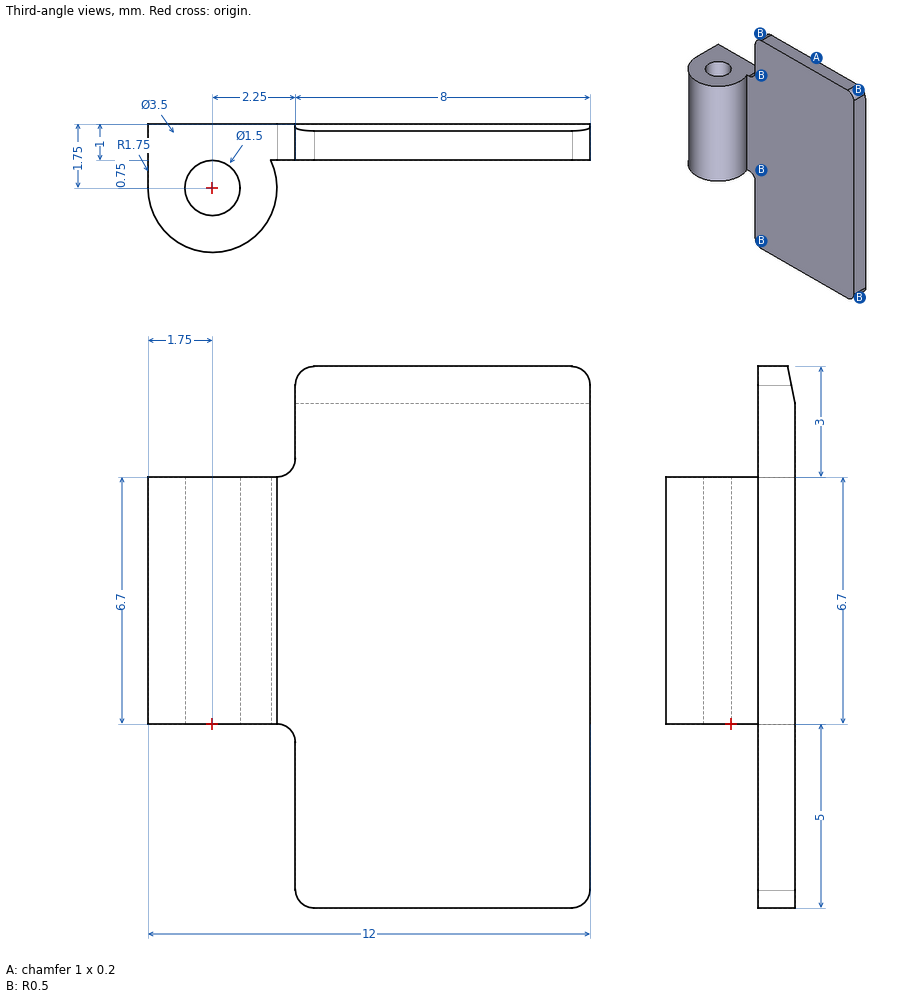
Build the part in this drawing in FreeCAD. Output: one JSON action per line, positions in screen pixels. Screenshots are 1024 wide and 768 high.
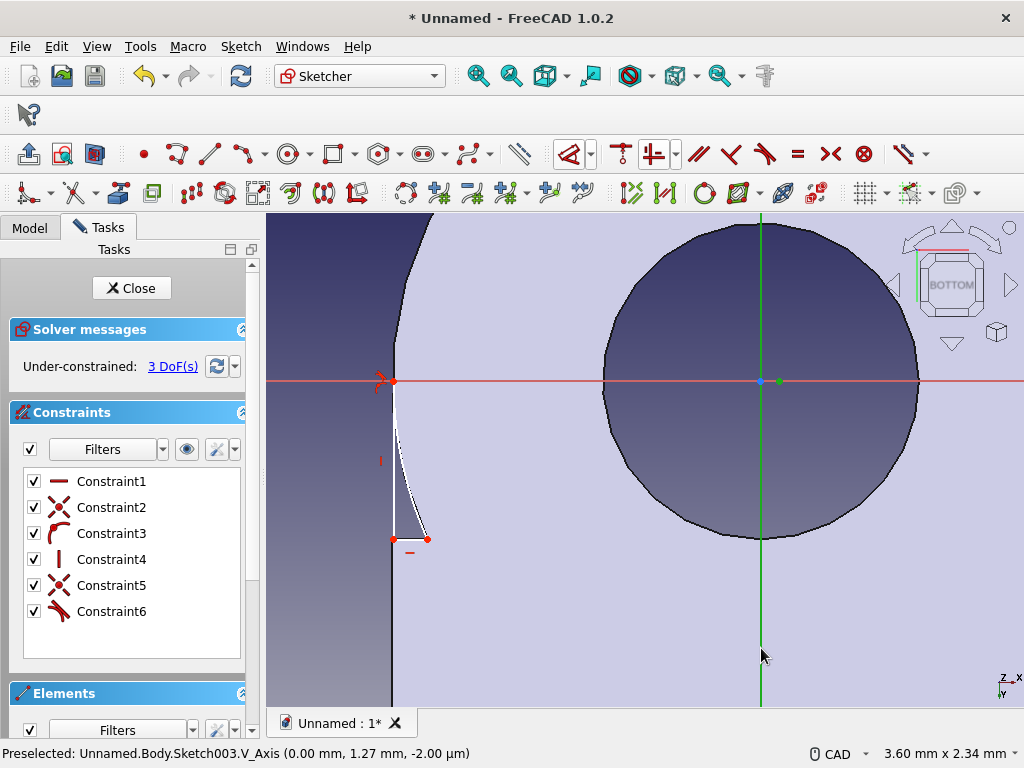
{"action": "key", "text": "c"}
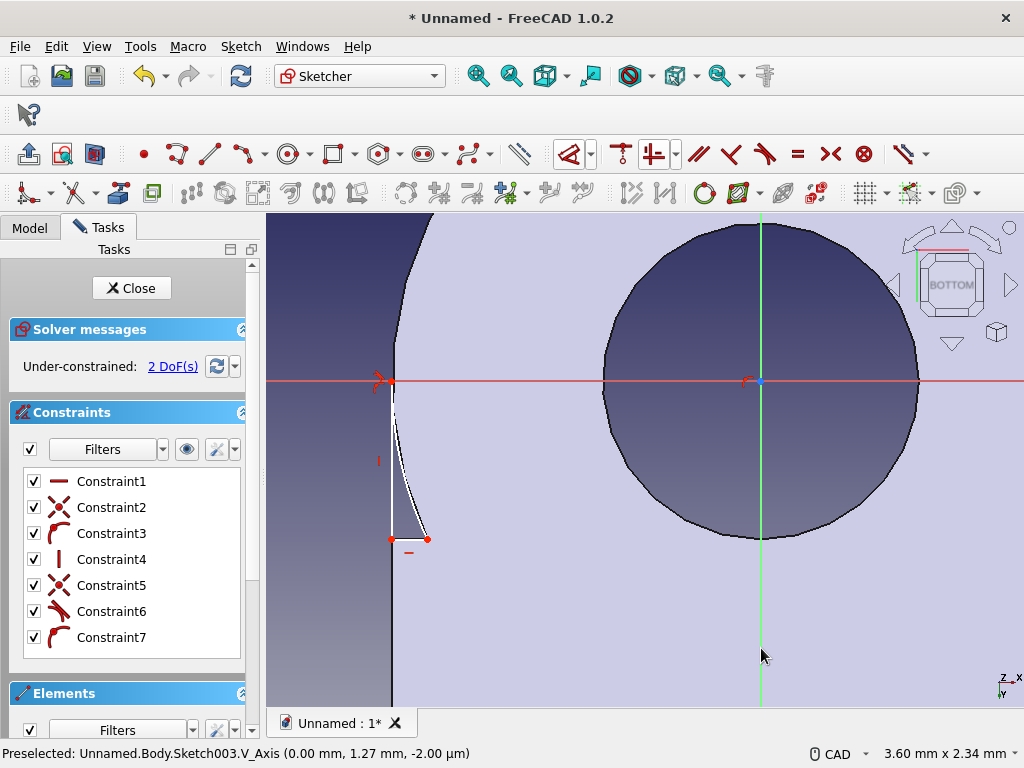
{"action": "left_click", "coordinate": [410, 494]}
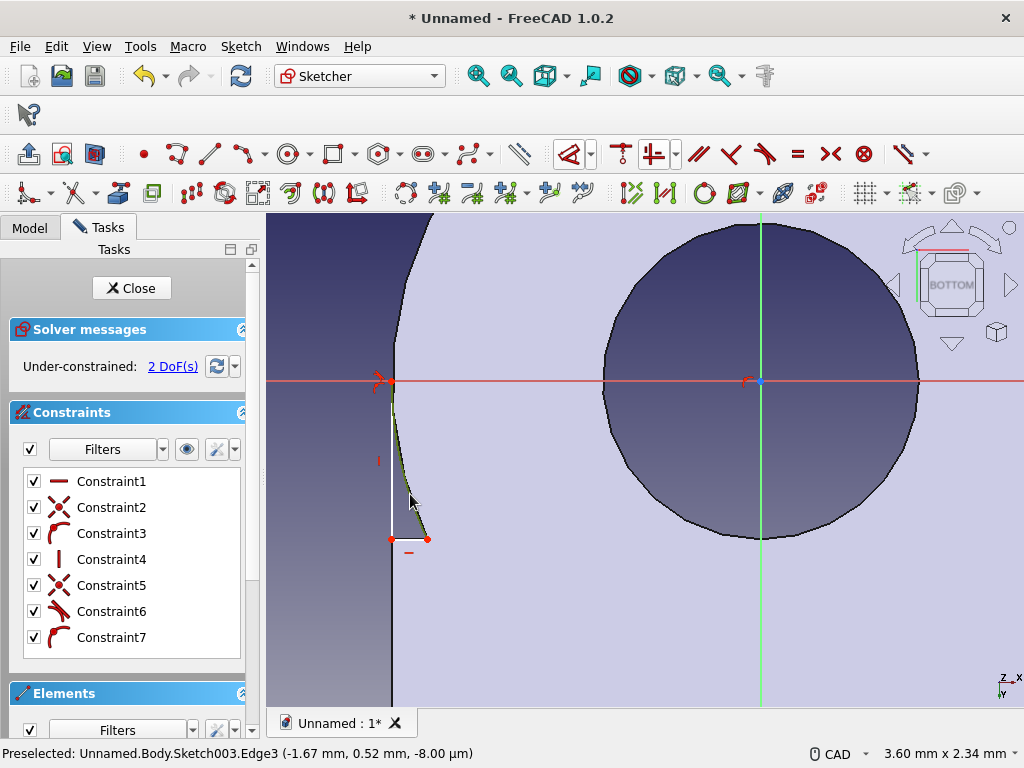
{"action": "key", "text": "k r"}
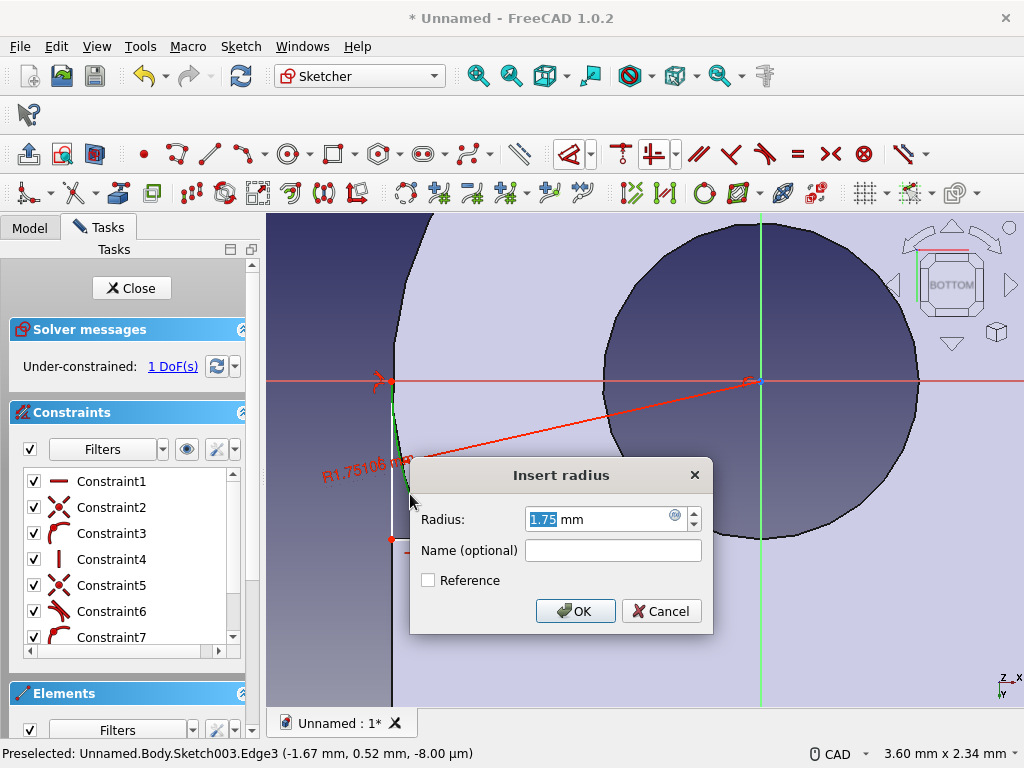
{"action": "type", "text": "1.75"}
{"action": "key", "text": "Return"}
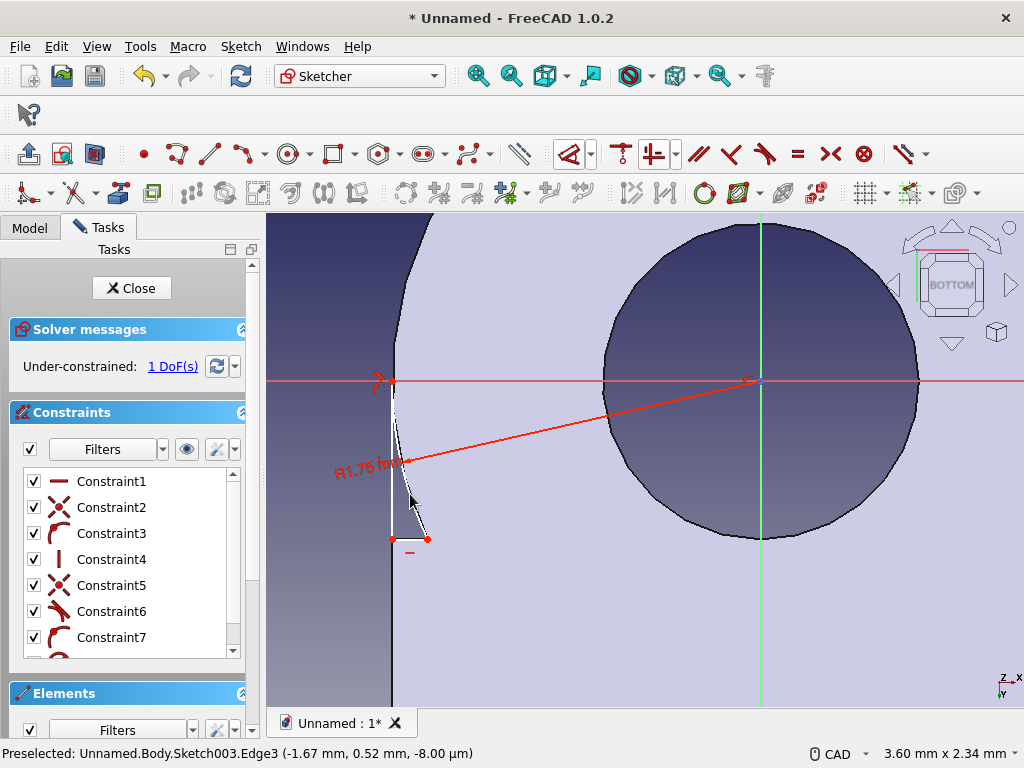
{"action": "left_click", "coordinate": [392, 492]}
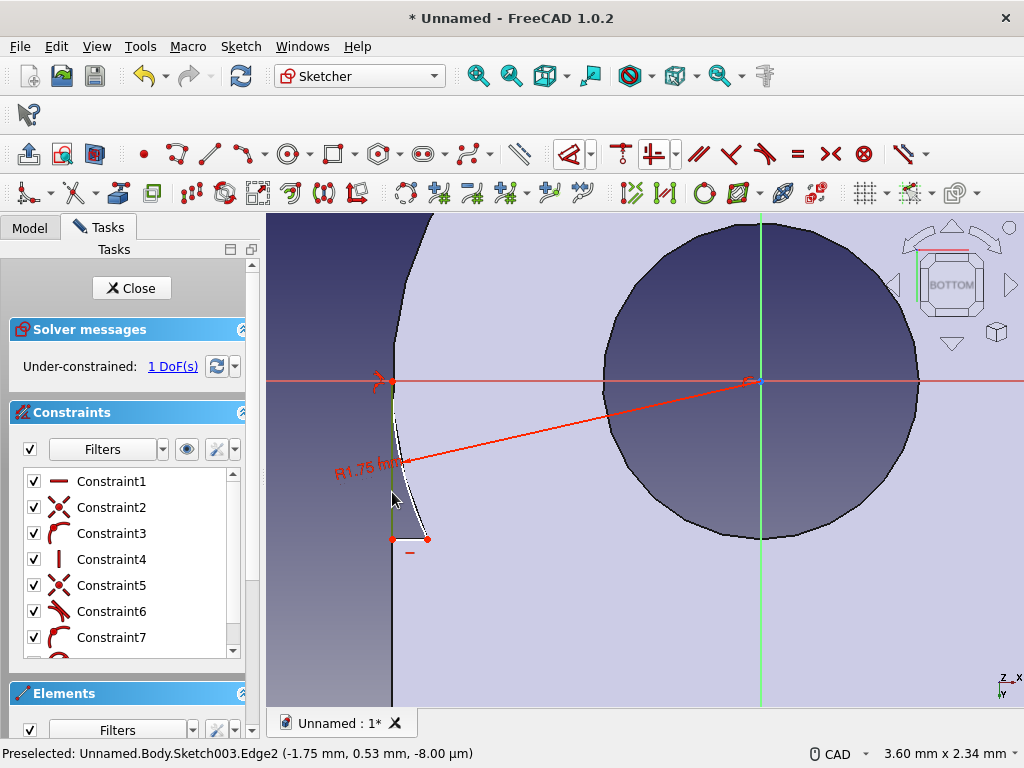
{"action": "left_click", "coordinate": [590, 154]}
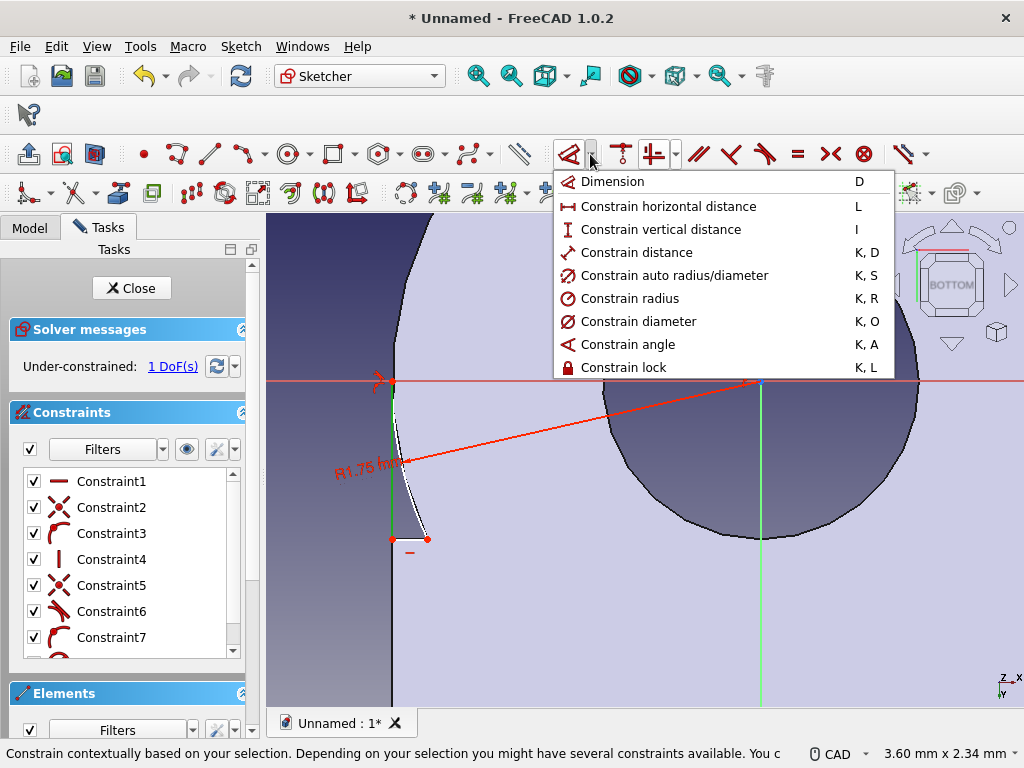
{"action": "left_click", "coordinate": [724, 230]}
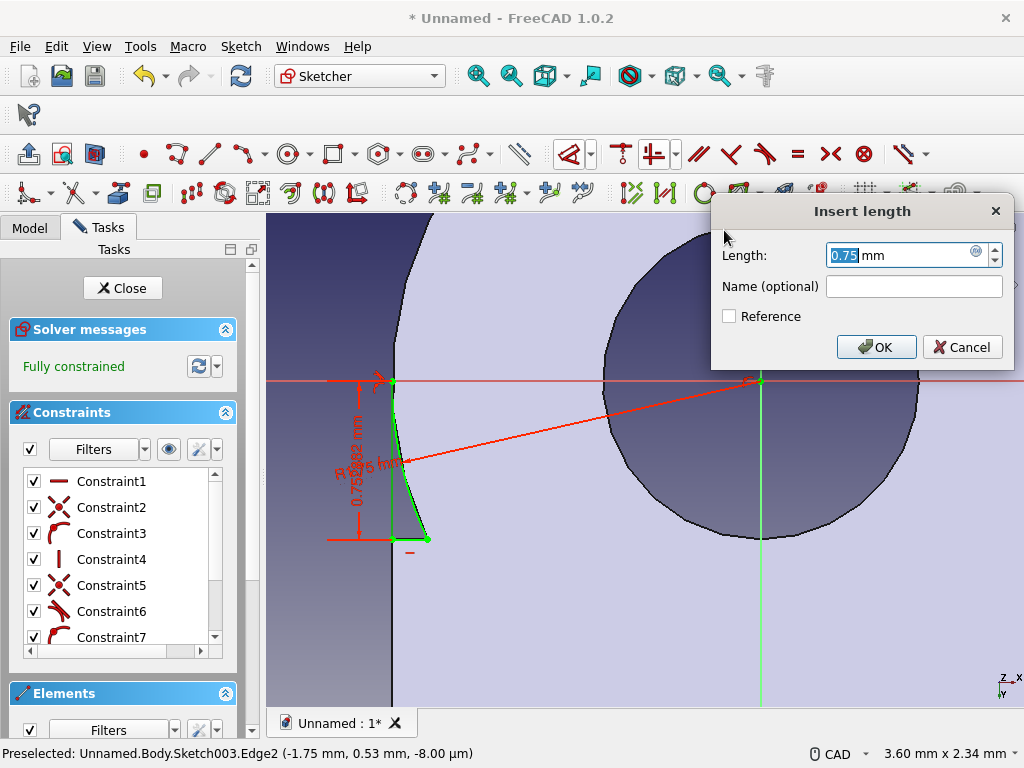
{"action": "type", "text": "0.75"}
{"action": "key", "text": "Return"}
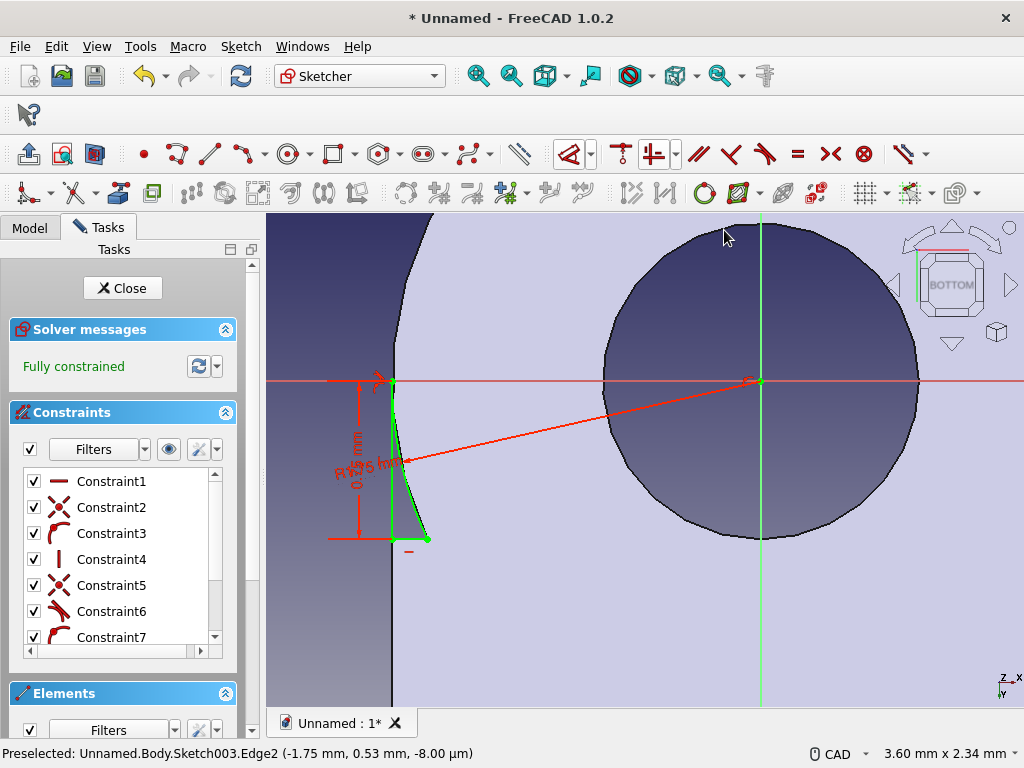
{"action": "left_click", "coordinate": [123, 288]}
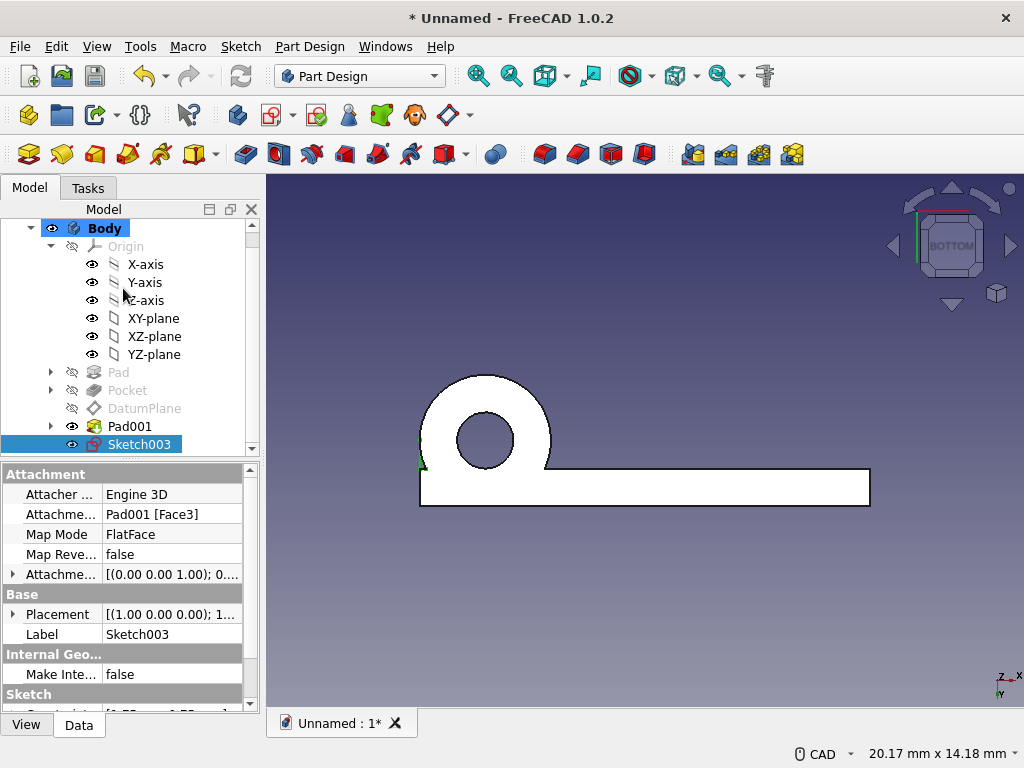
{"action": "left_click", "coordinate": [29, 154]}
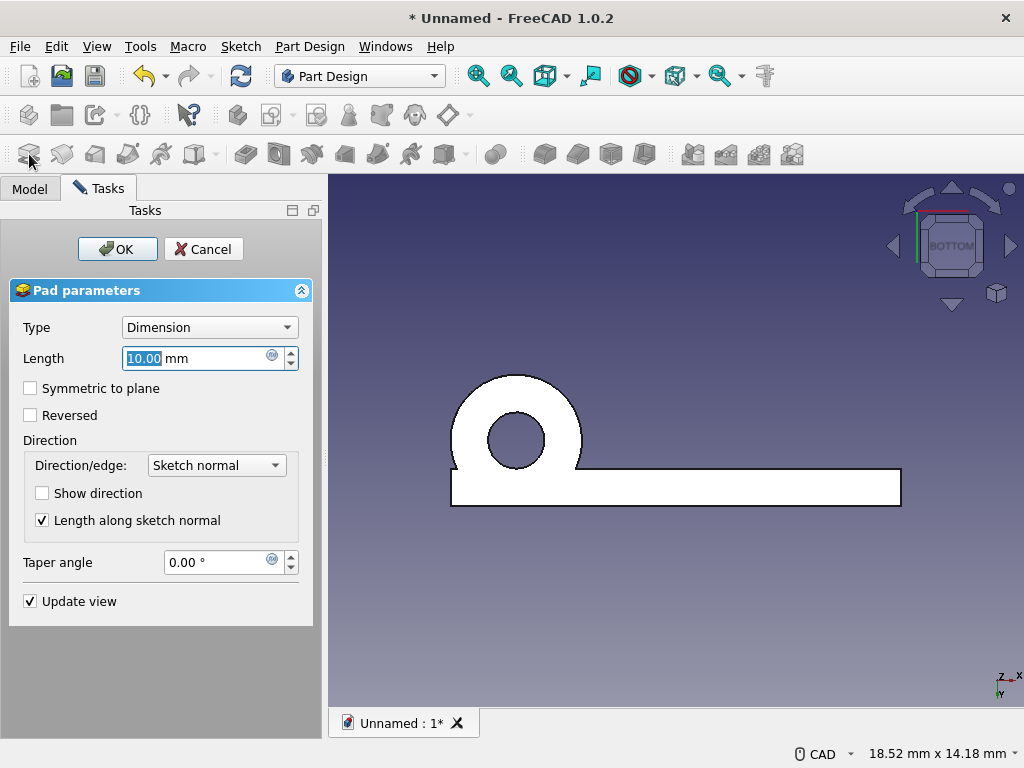
{"action": "type", "text": "6.7"}
{"action": "key", "text": "Tab"}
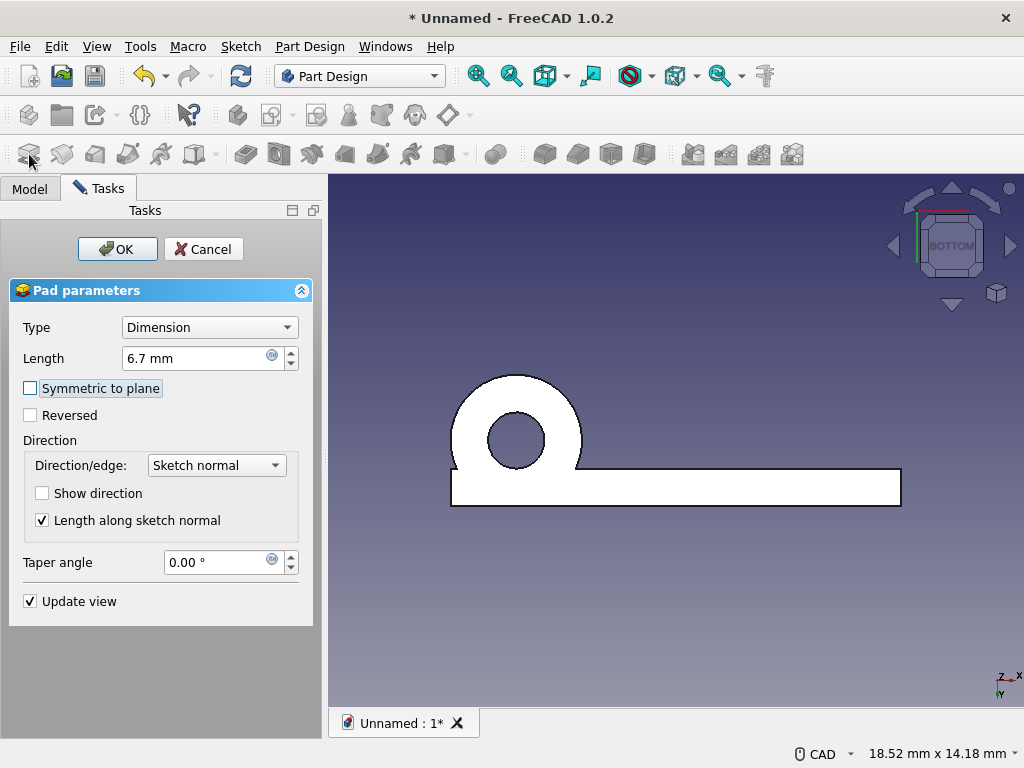
{"action": "left_click", "coordinate": [31, 415]}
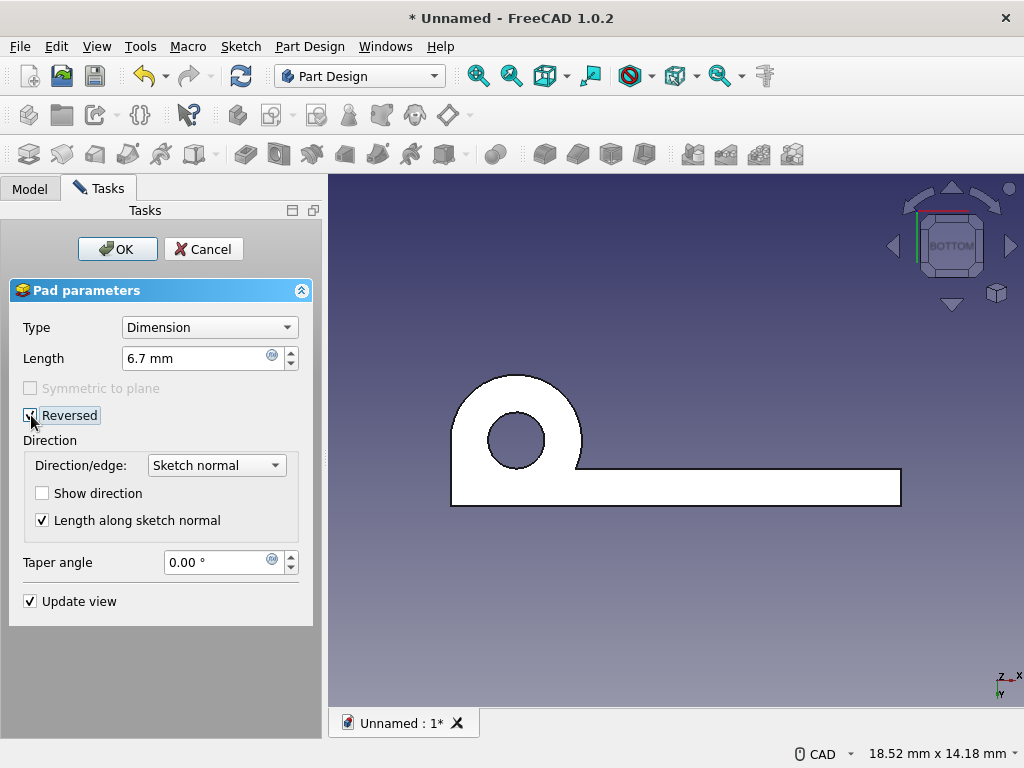
{"action": "left_click", "coordinate": [118, 249]}